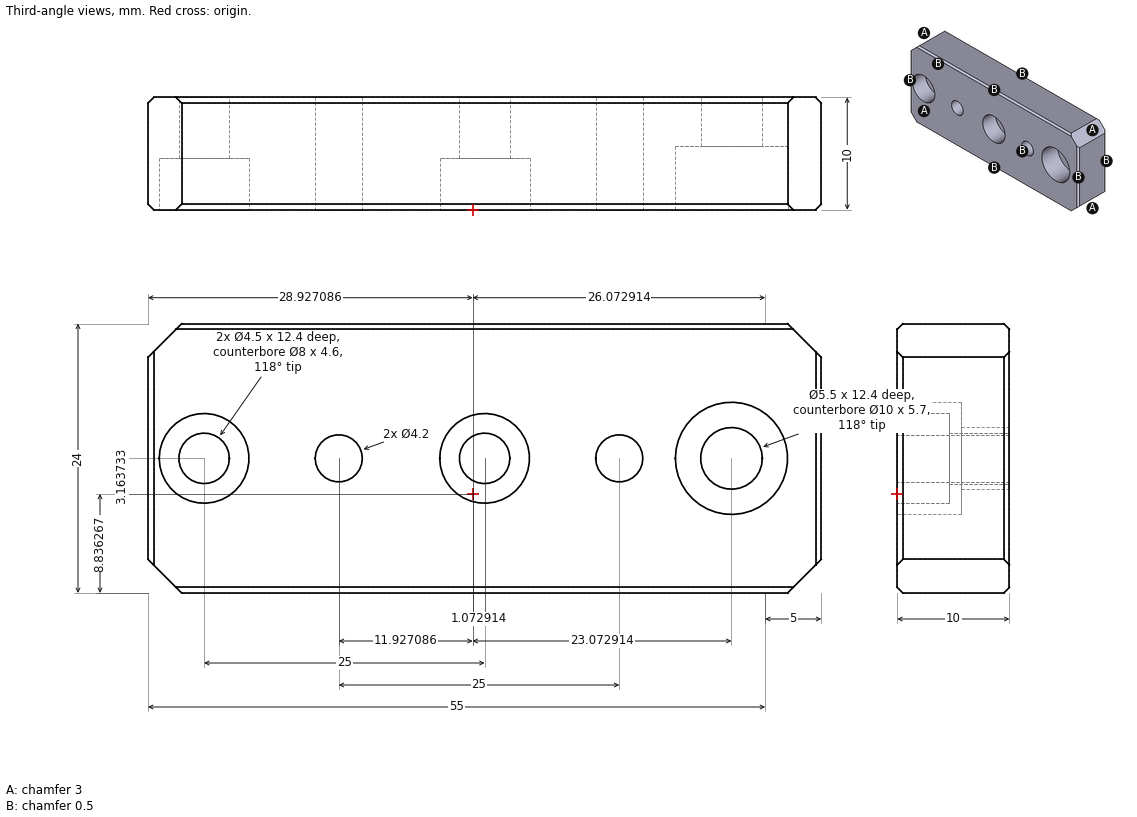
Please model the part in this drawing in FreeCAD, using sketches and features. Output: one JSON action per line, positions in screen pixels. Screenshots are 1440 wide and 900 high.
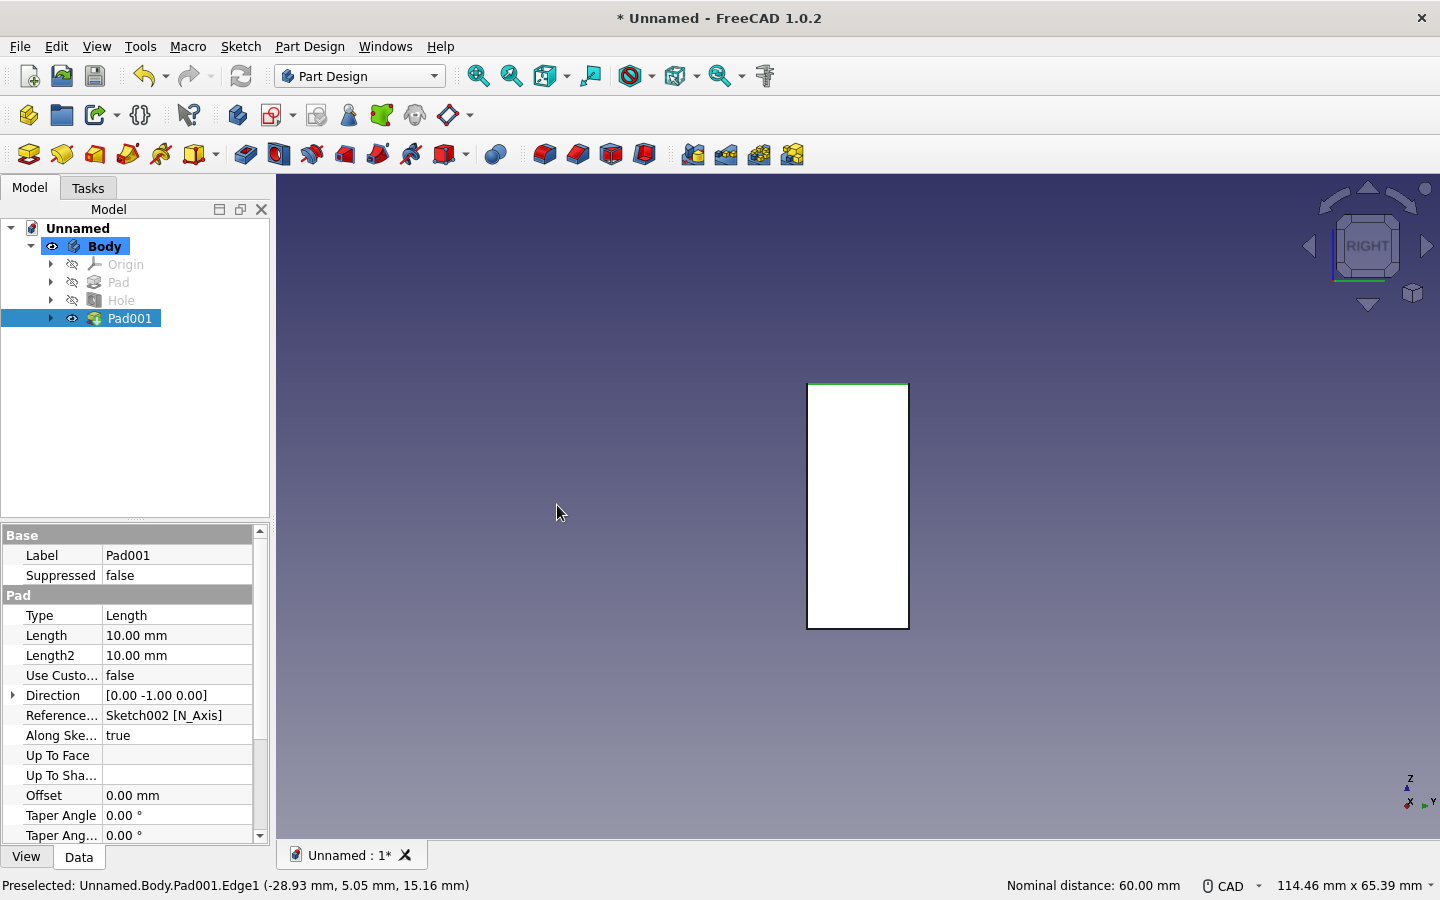
{"action": "left_click", "coordinate": [858, 628], "text": "ctrl"}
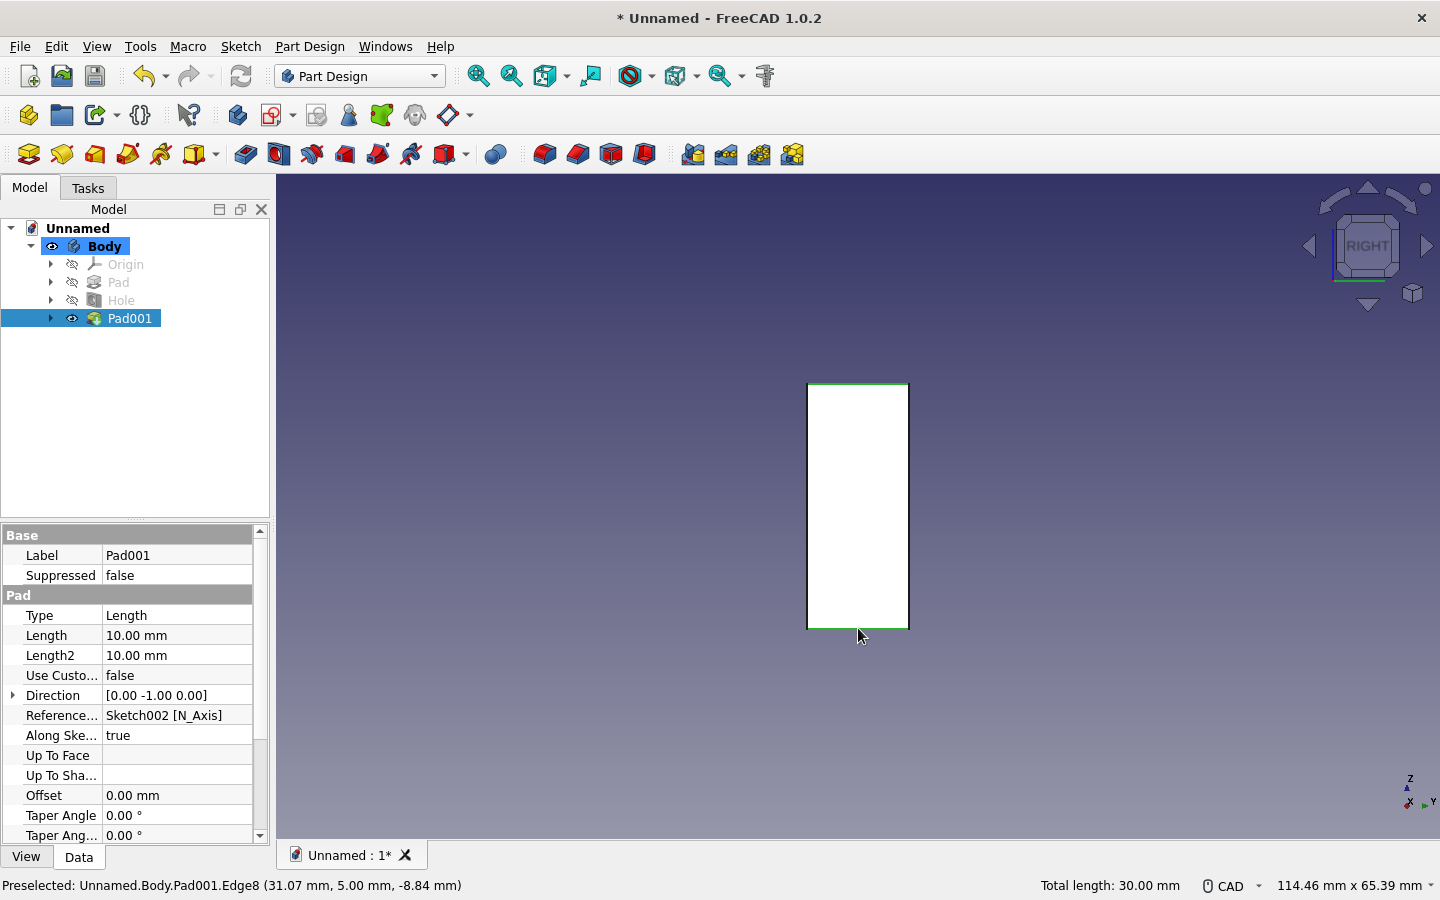
{"action": "key", "text": "5"}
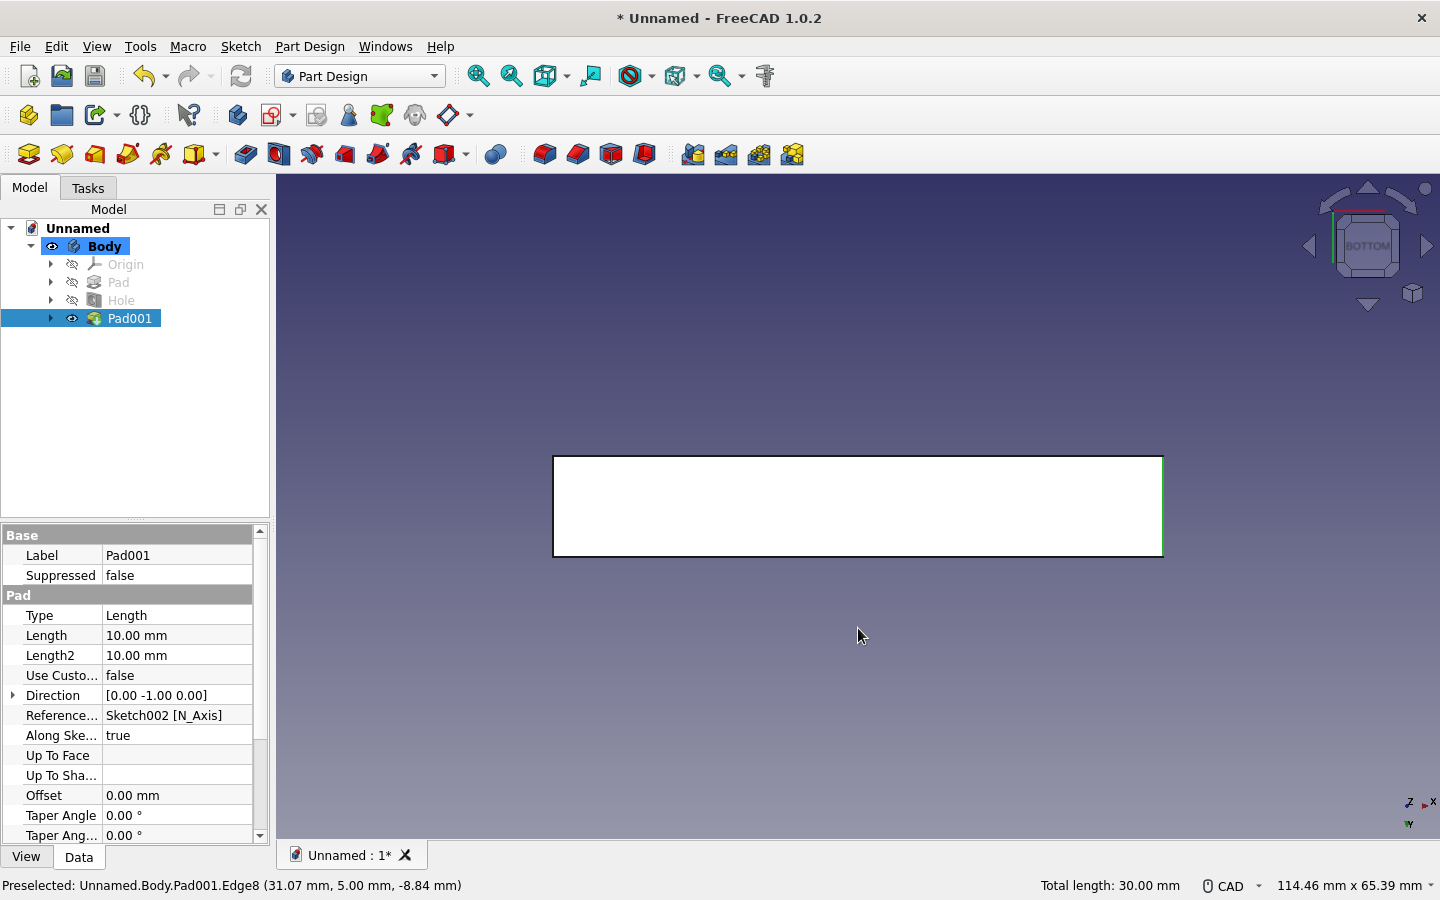
{"action": "left_click", "coordinate": [553, 505], "text": "ctrl"}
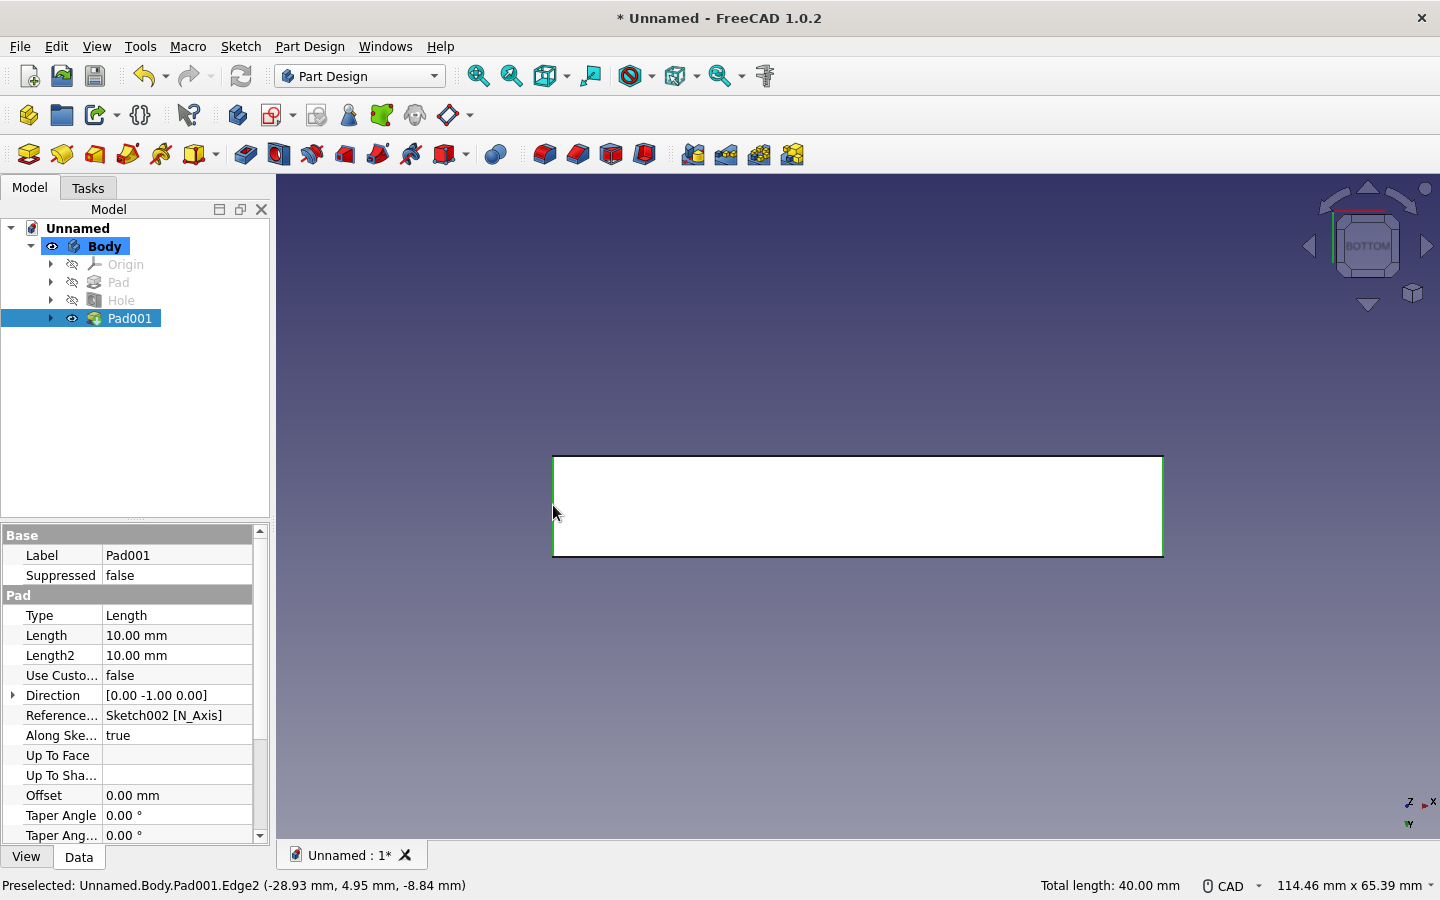
{"action": "left_click", "coordinate": [578, 154]}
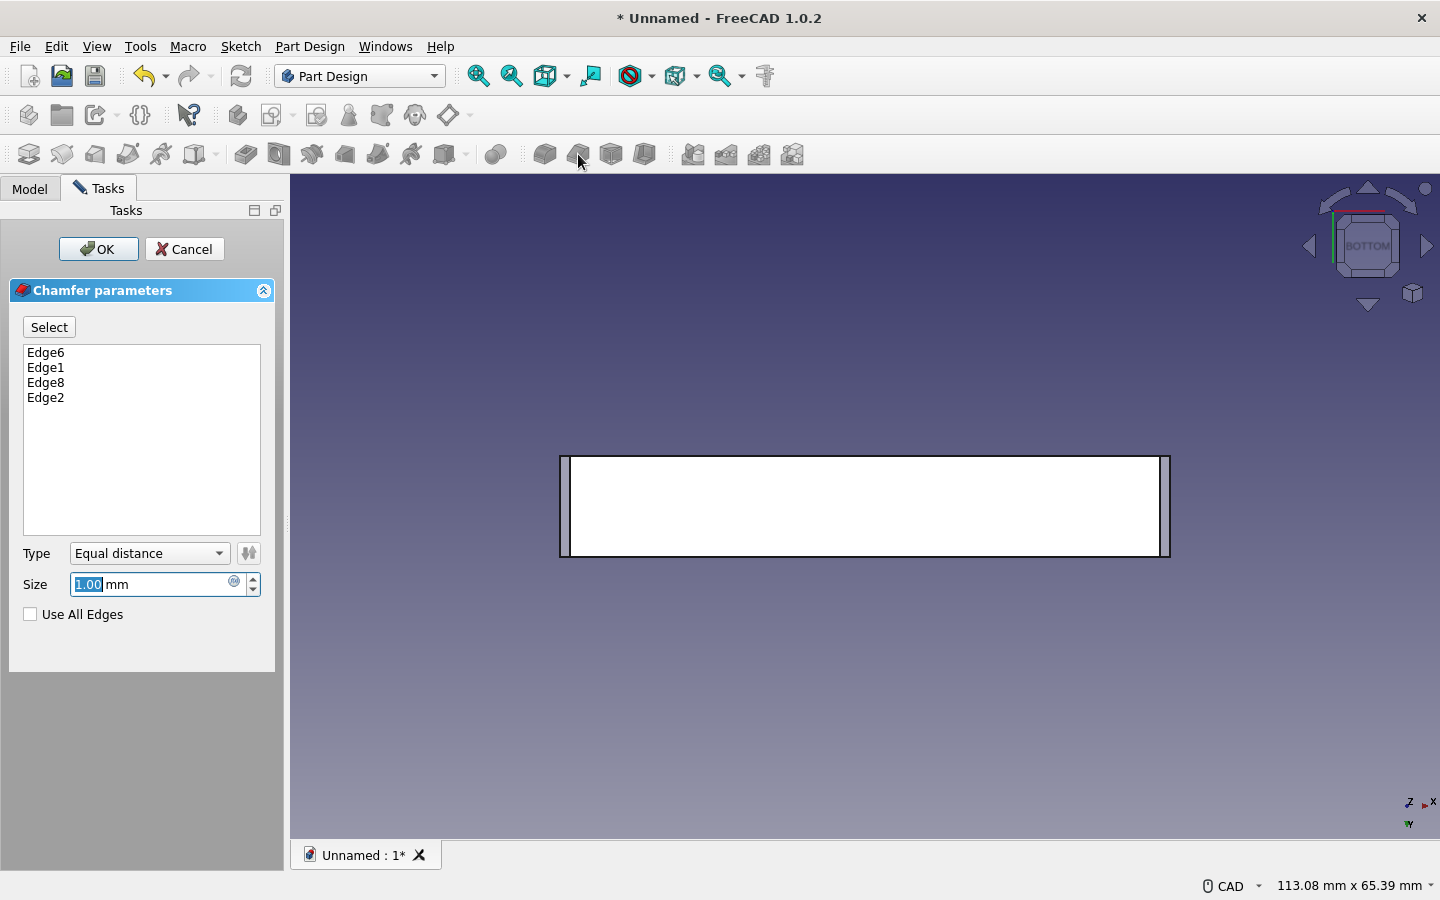
{"action": "type", "text": "3"}
{"action": "key", "text": "Tab"}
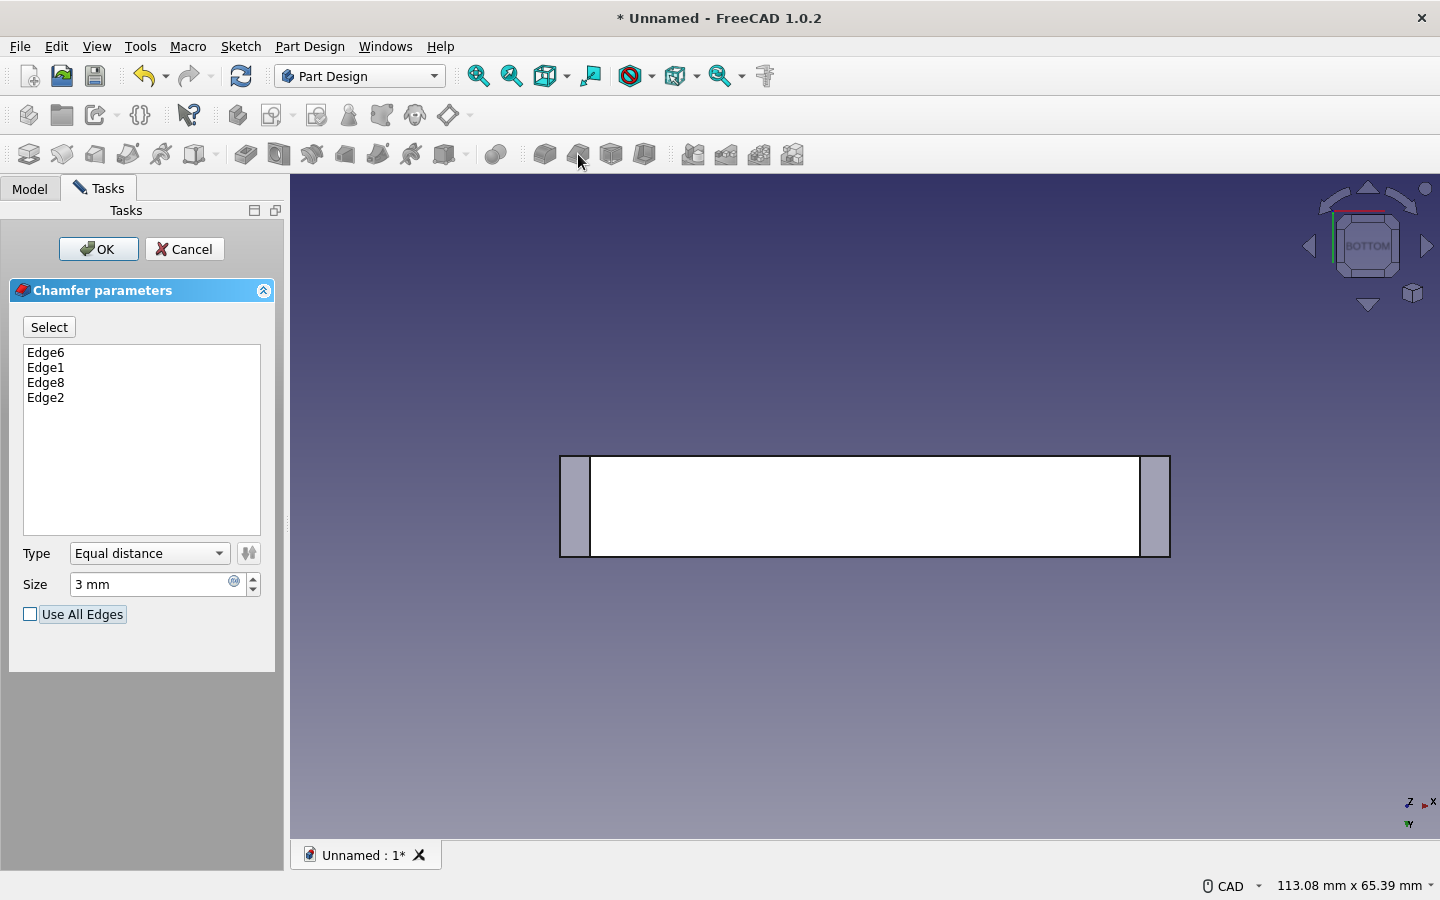
{"action": "left_click", "coordinate": [99, 249]}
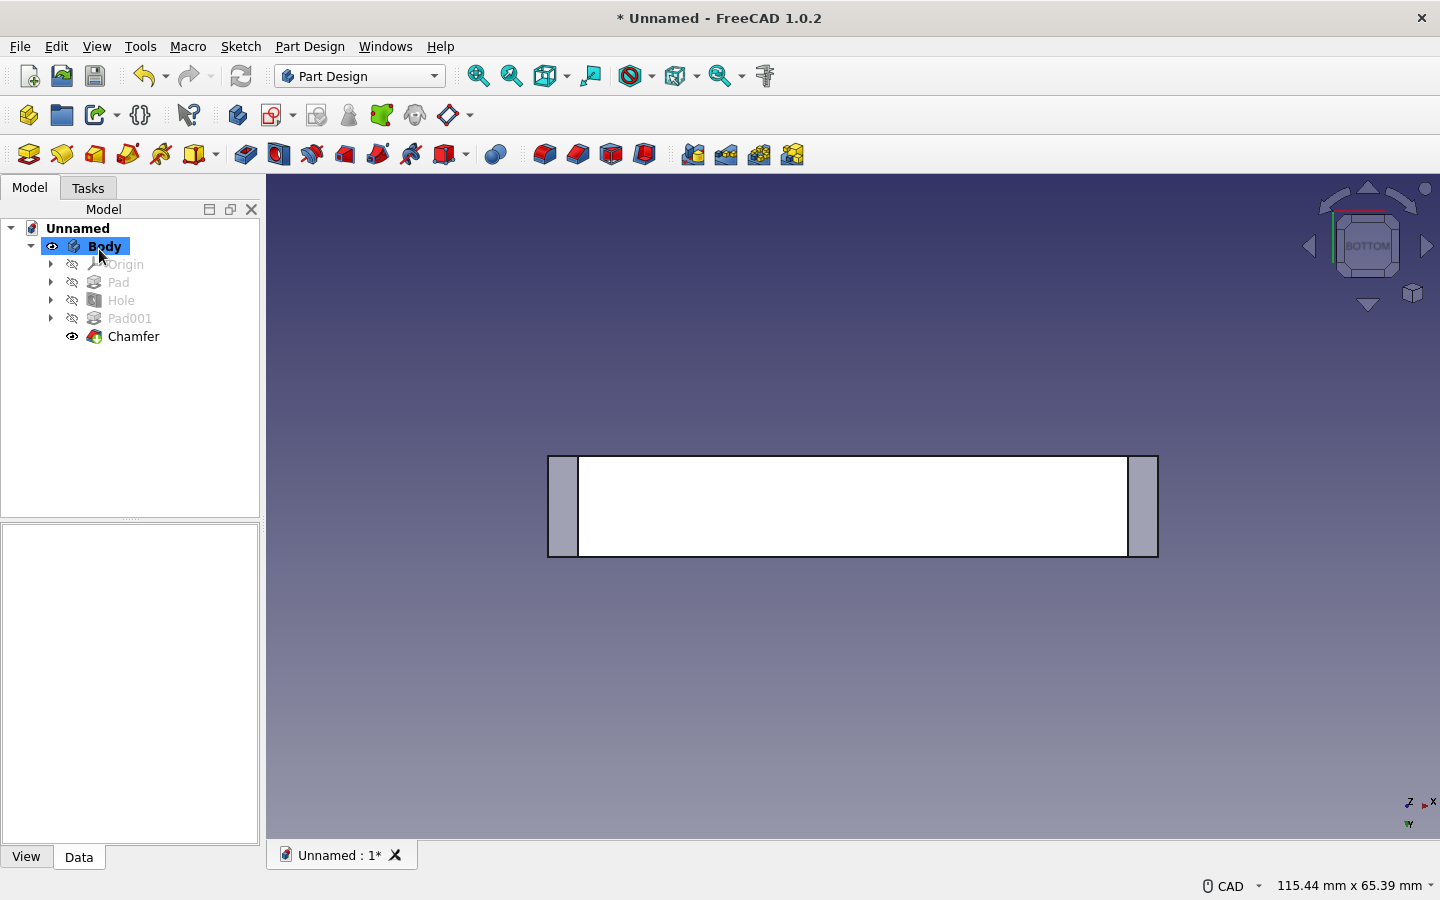
{"action": "left_click", "coordinate": [853, 455]}